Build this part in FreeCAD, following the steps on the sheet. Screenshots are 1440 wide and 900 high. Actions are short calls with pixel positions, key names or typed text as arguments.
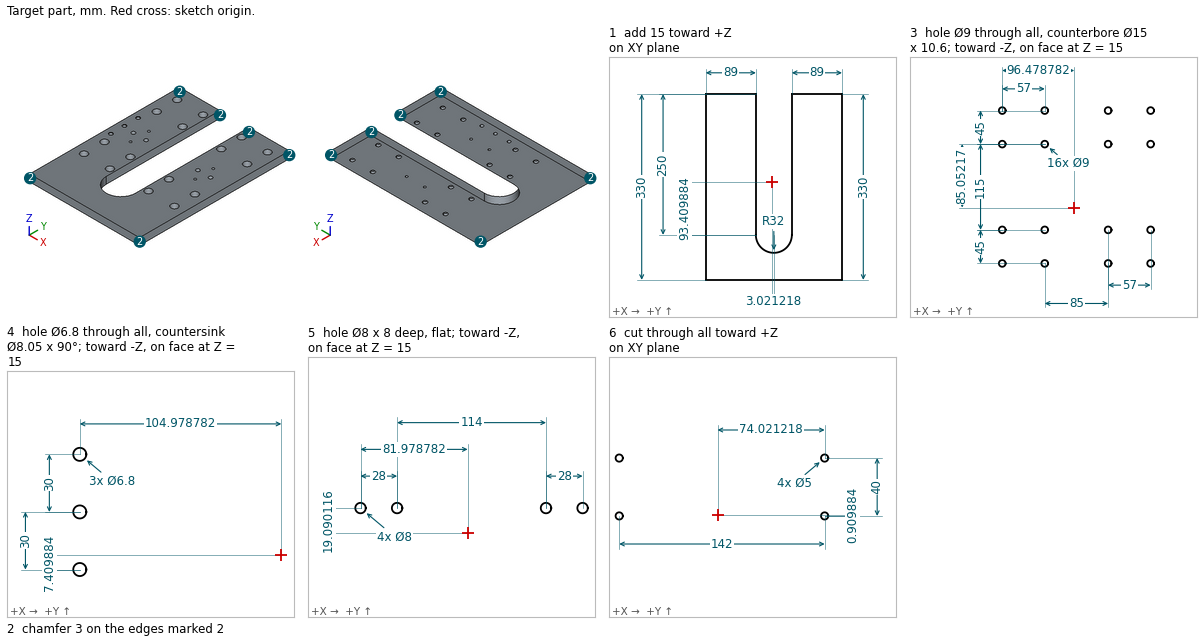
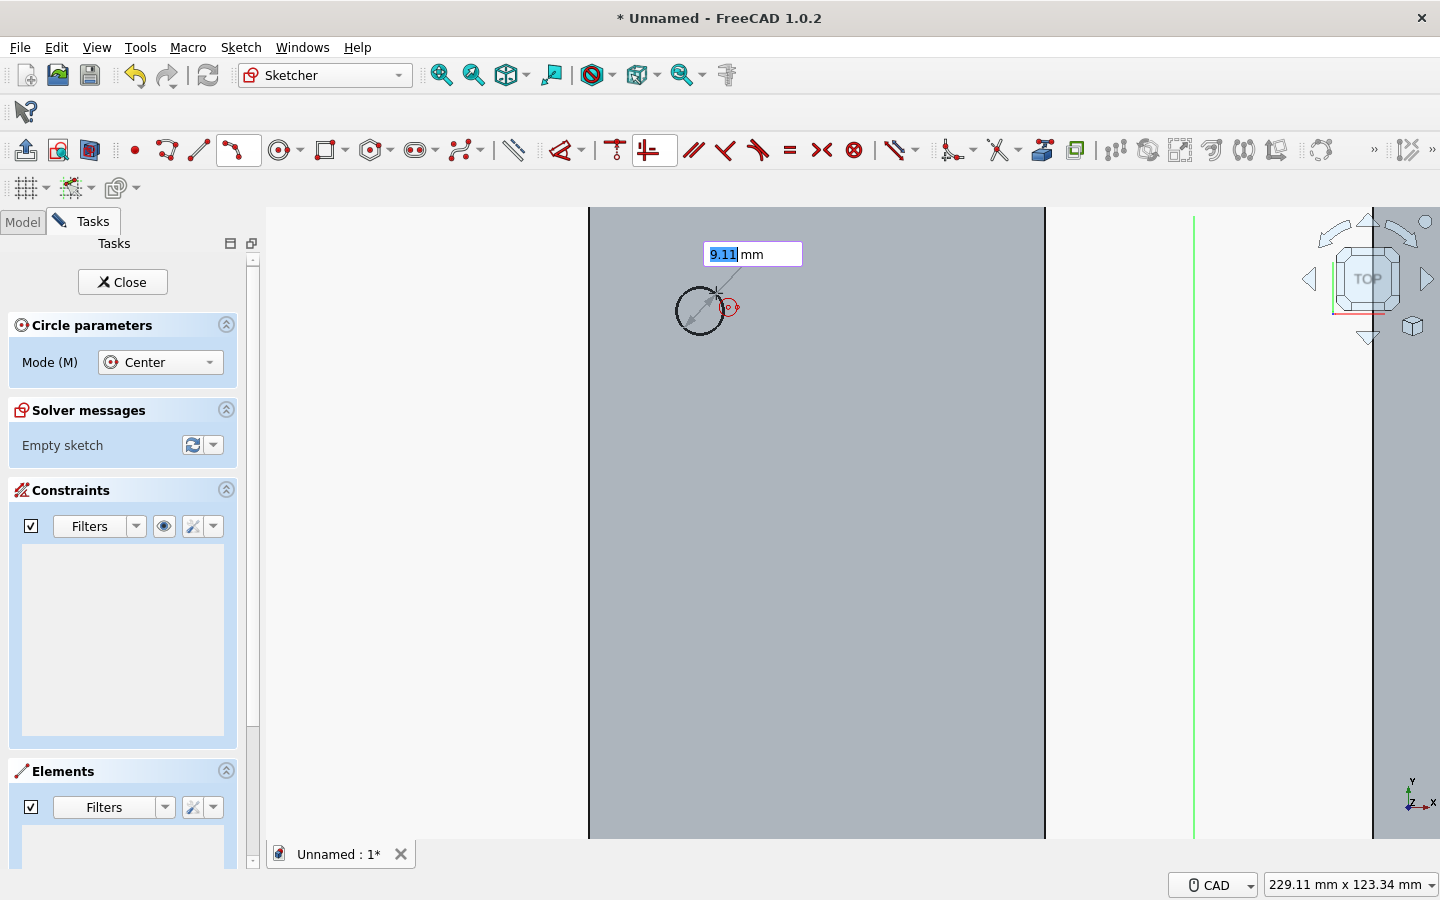
text(9)
key(Return)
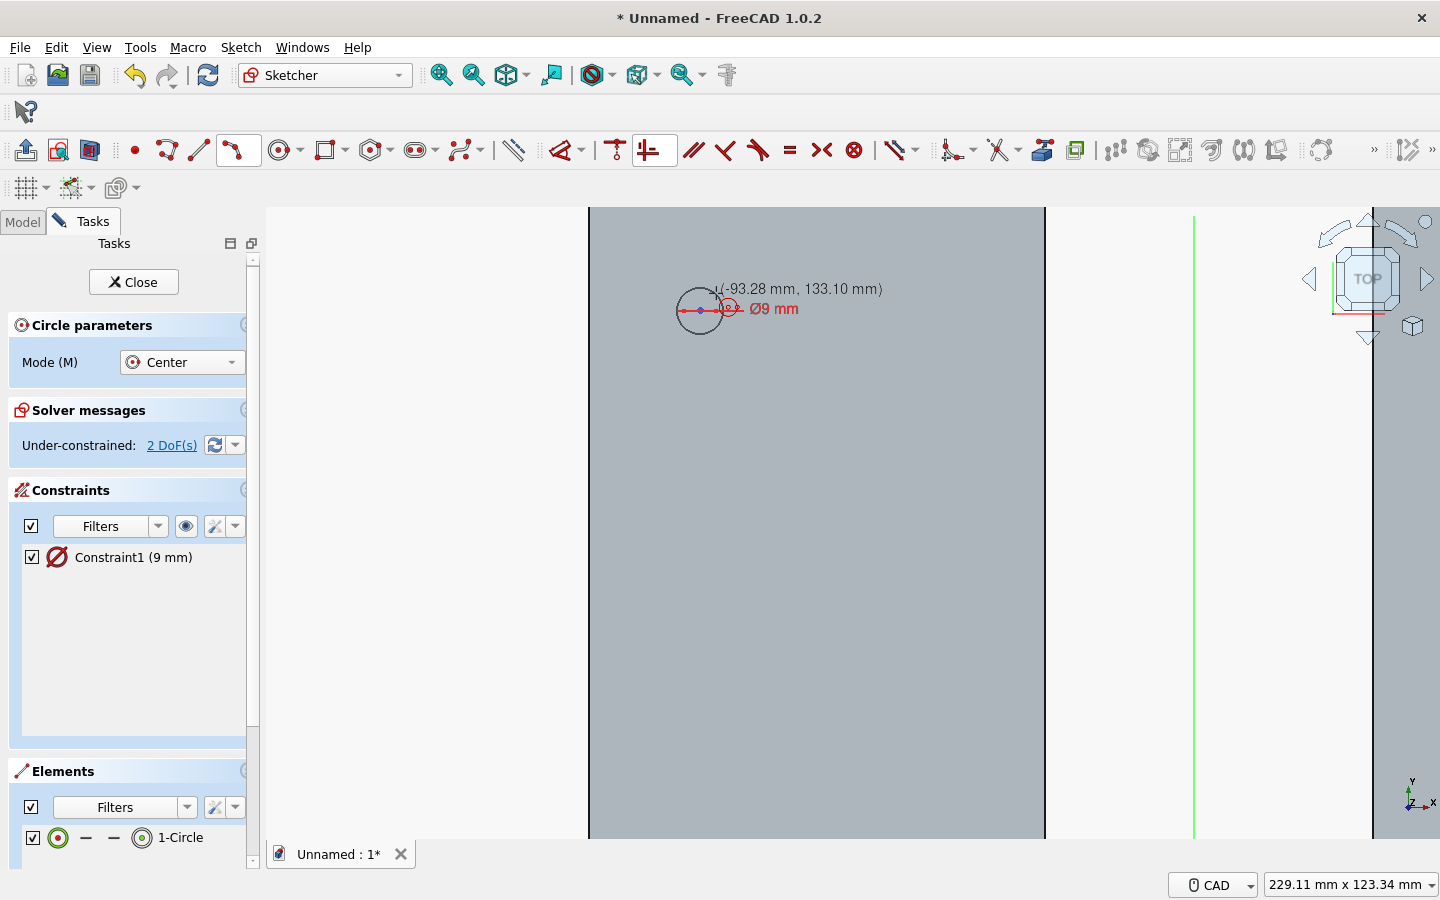
click(992, 310)
move(1008, 293)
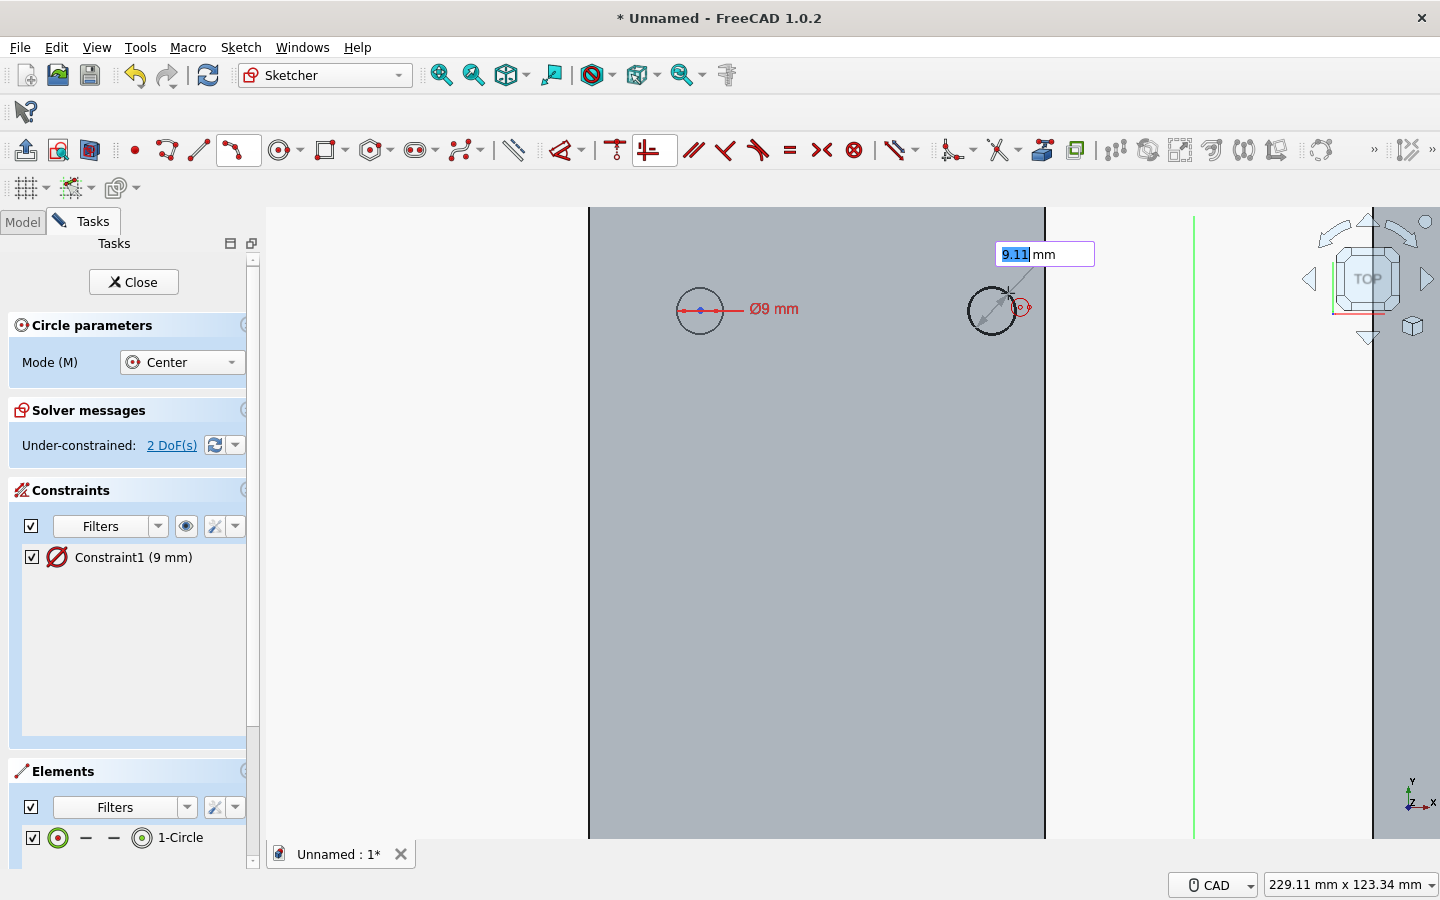
text(9)
key(Return)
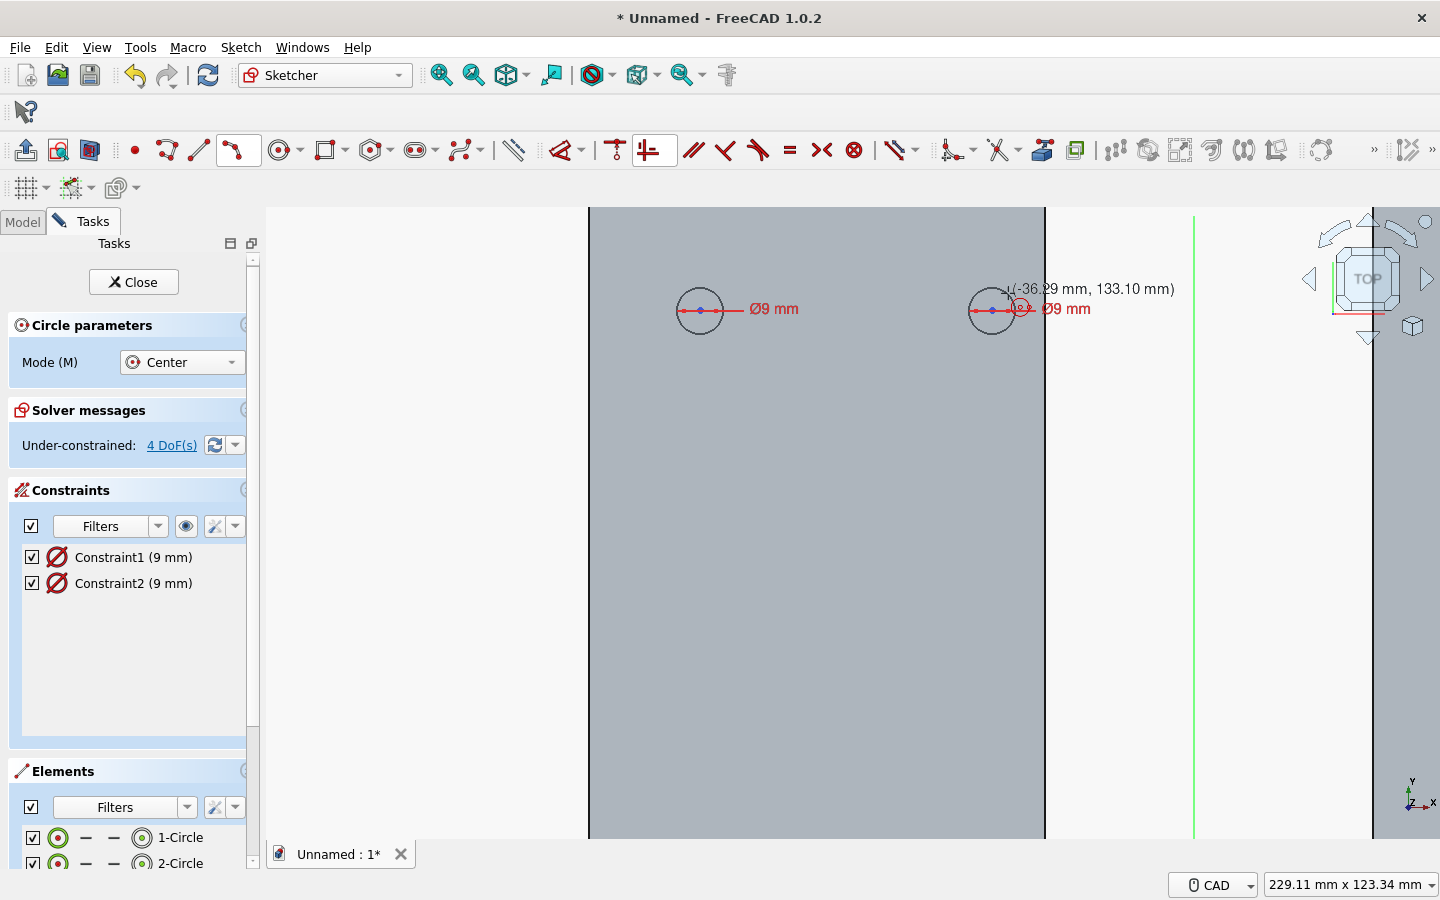
click(992, 540)
move(1008, 524)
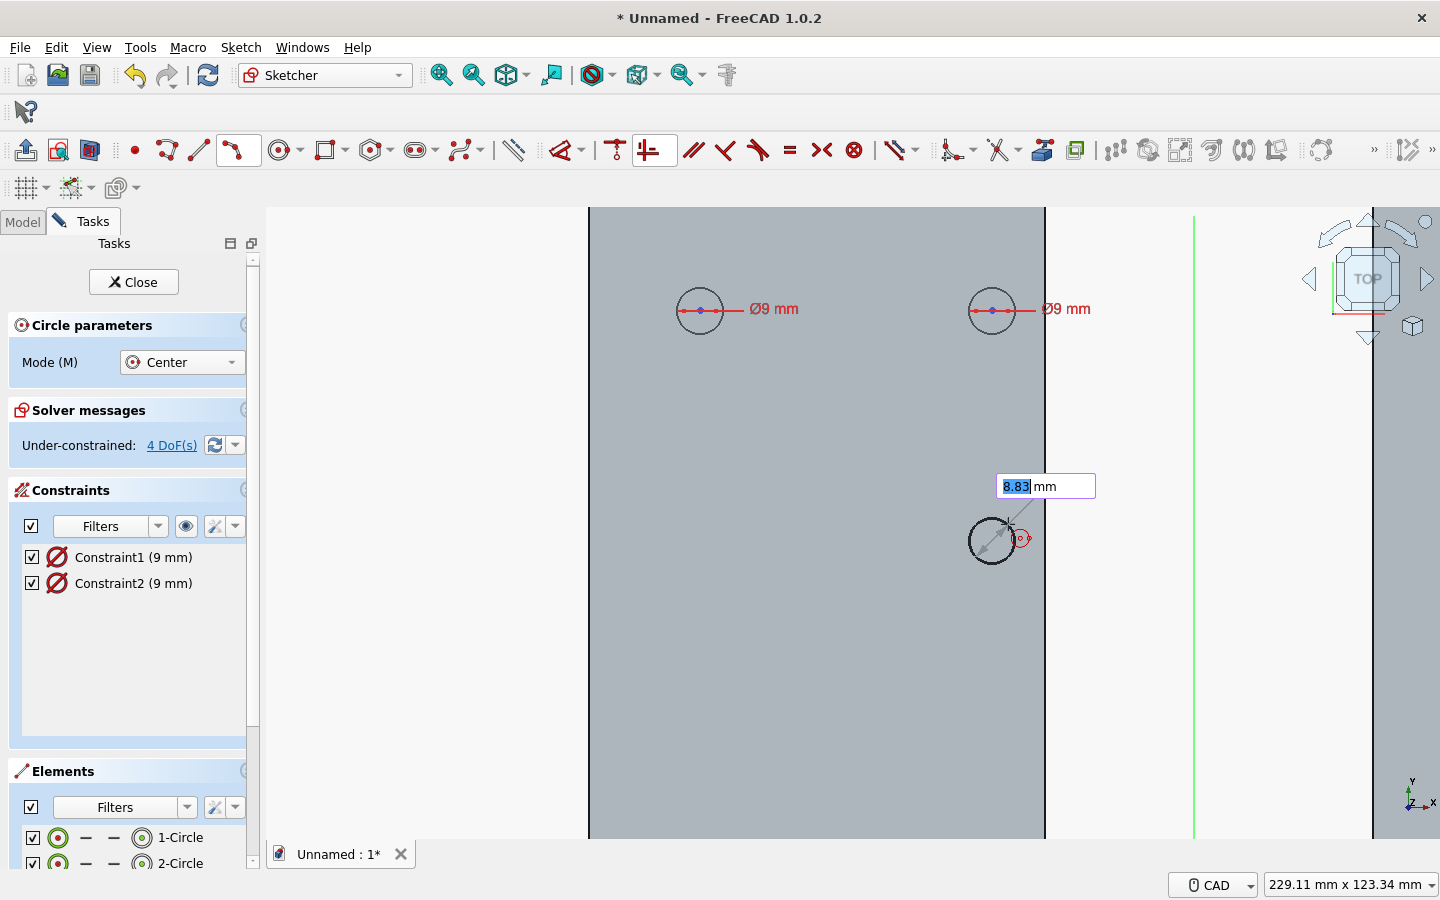
text(9)
key(Return)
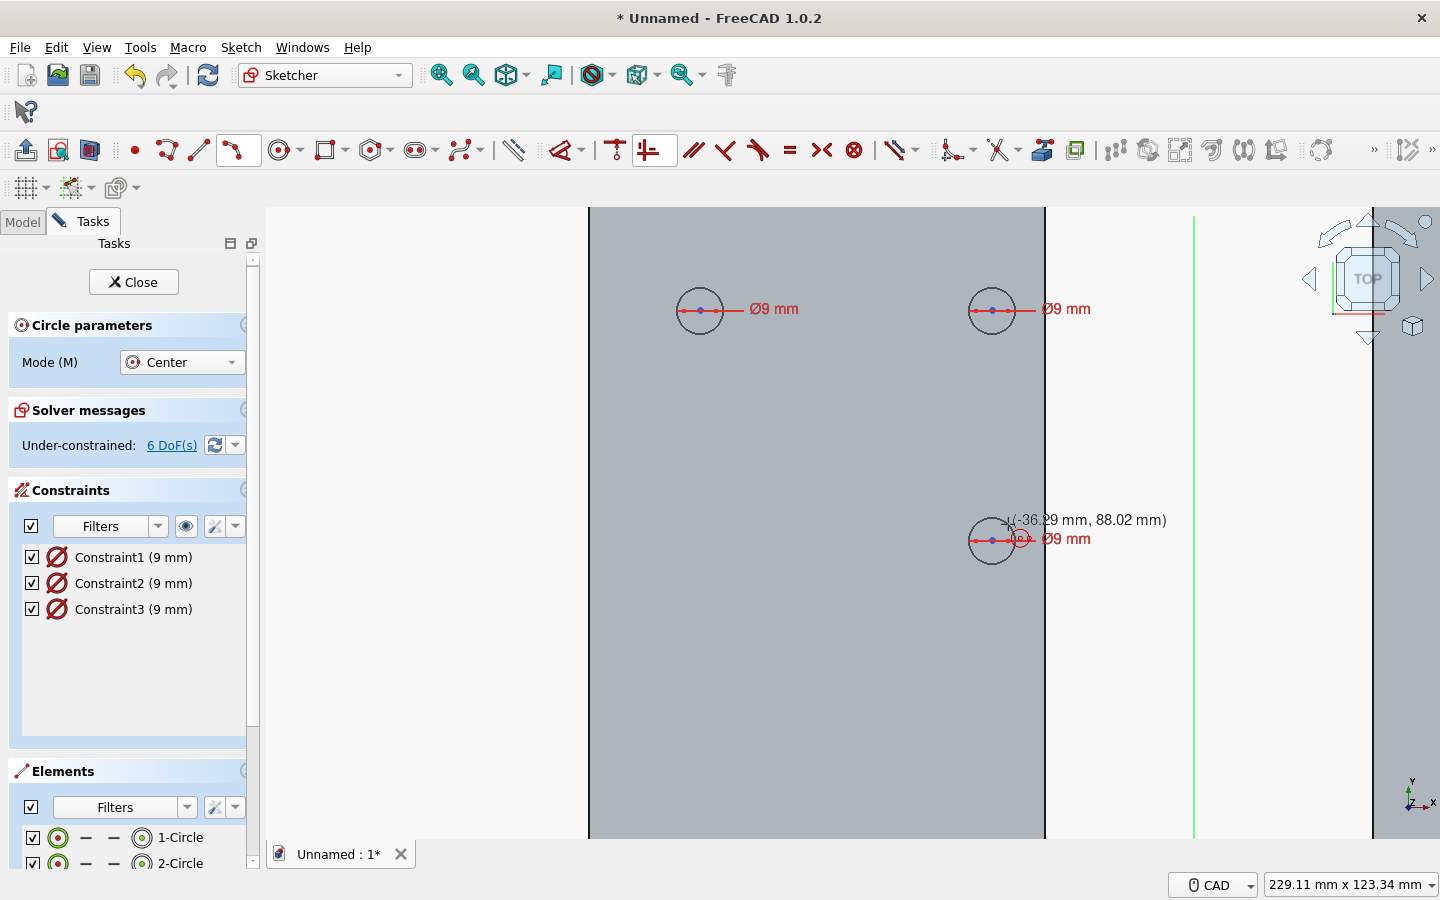
click(700, 540)
move(716, 524)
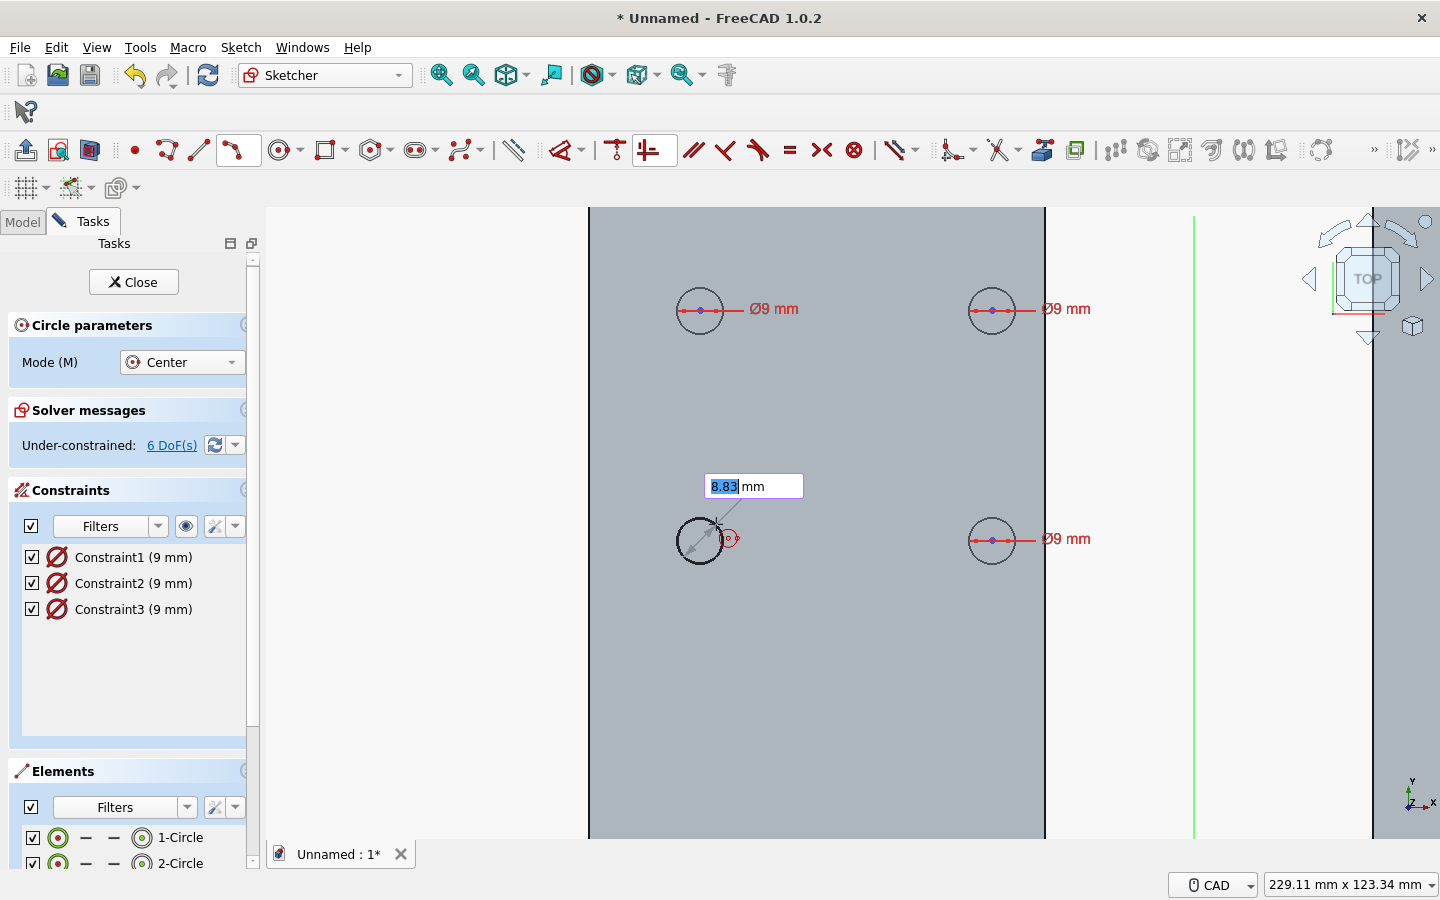
text(9)
key(Return)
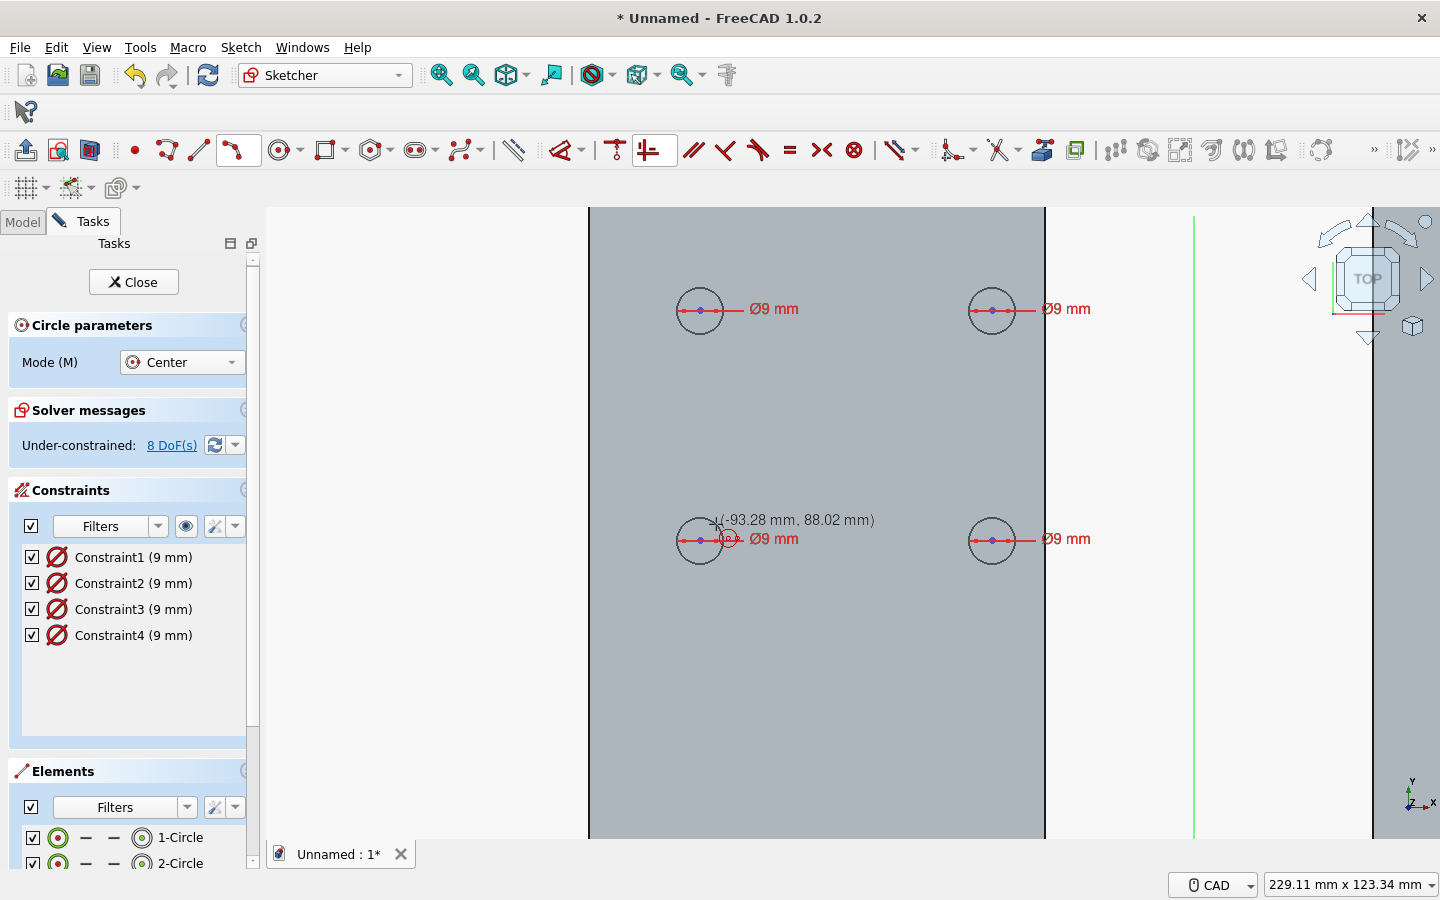
scroll(537, 342, down, 5)